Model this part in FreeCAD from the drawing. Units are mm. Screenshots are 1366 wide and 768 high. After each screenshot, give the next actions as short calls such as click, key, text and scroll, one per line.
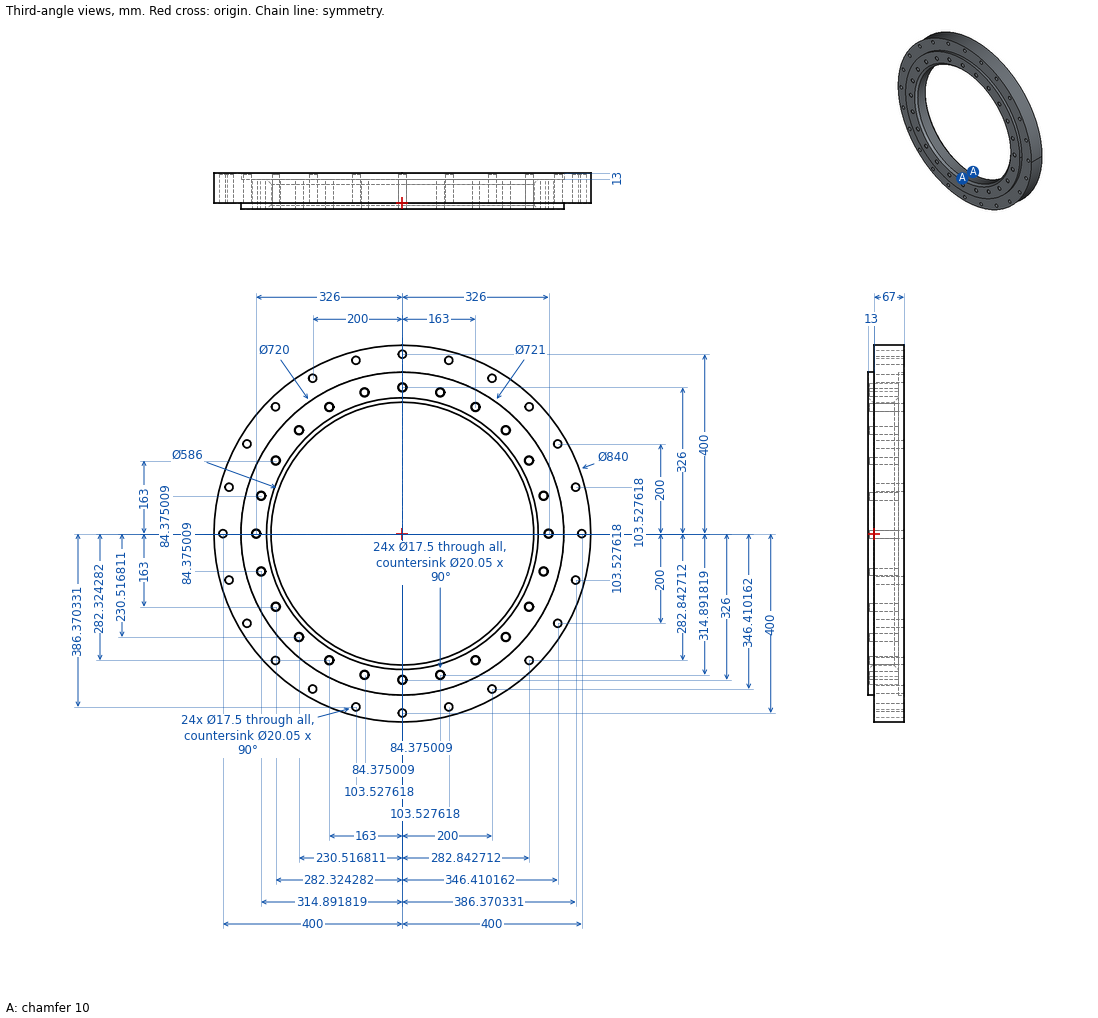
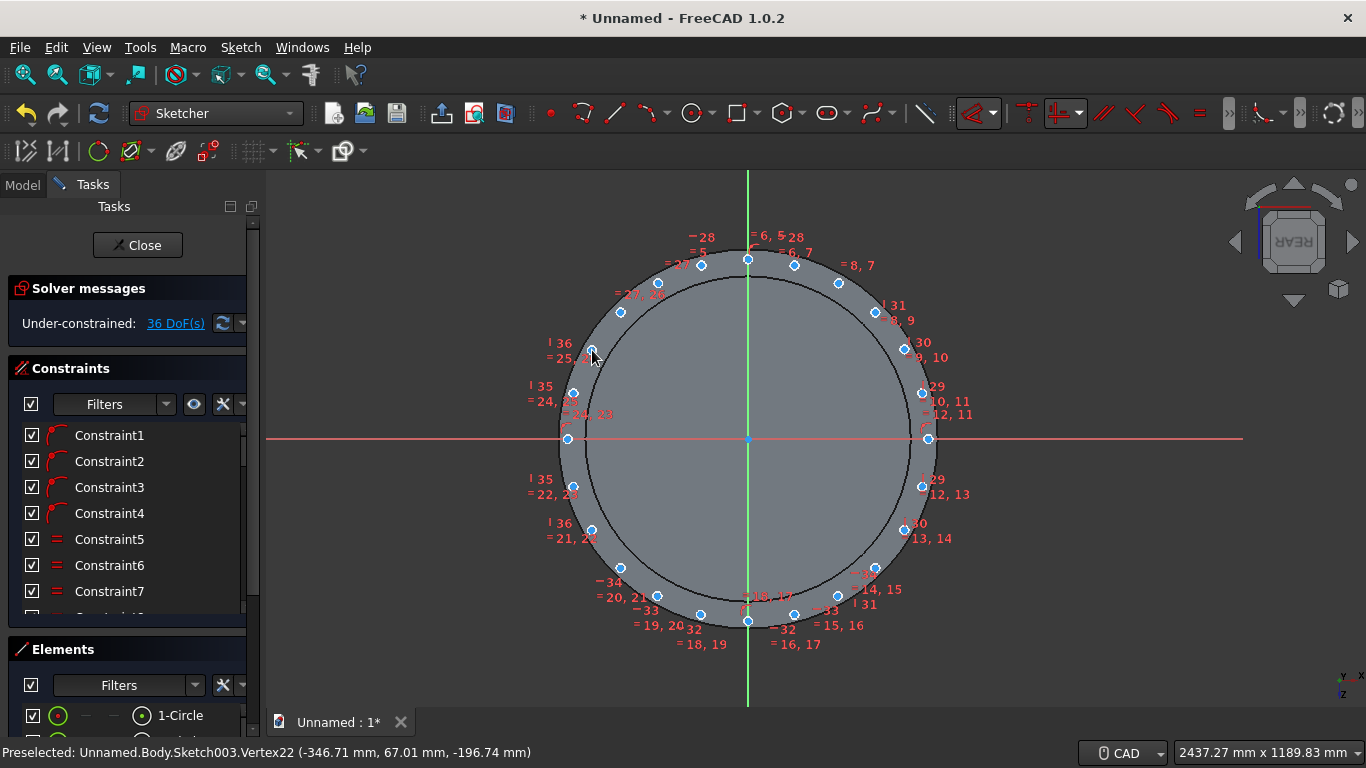
click(839, 283)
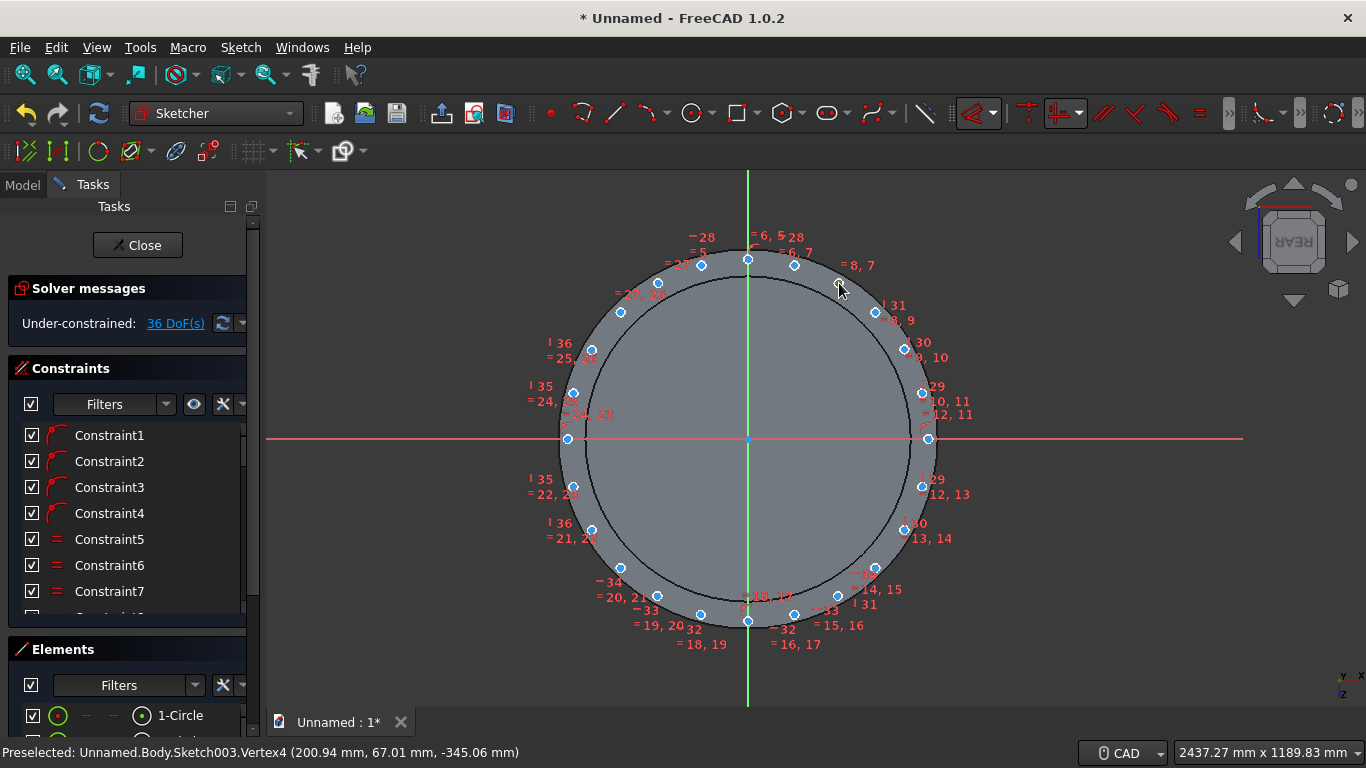
click(838, 596)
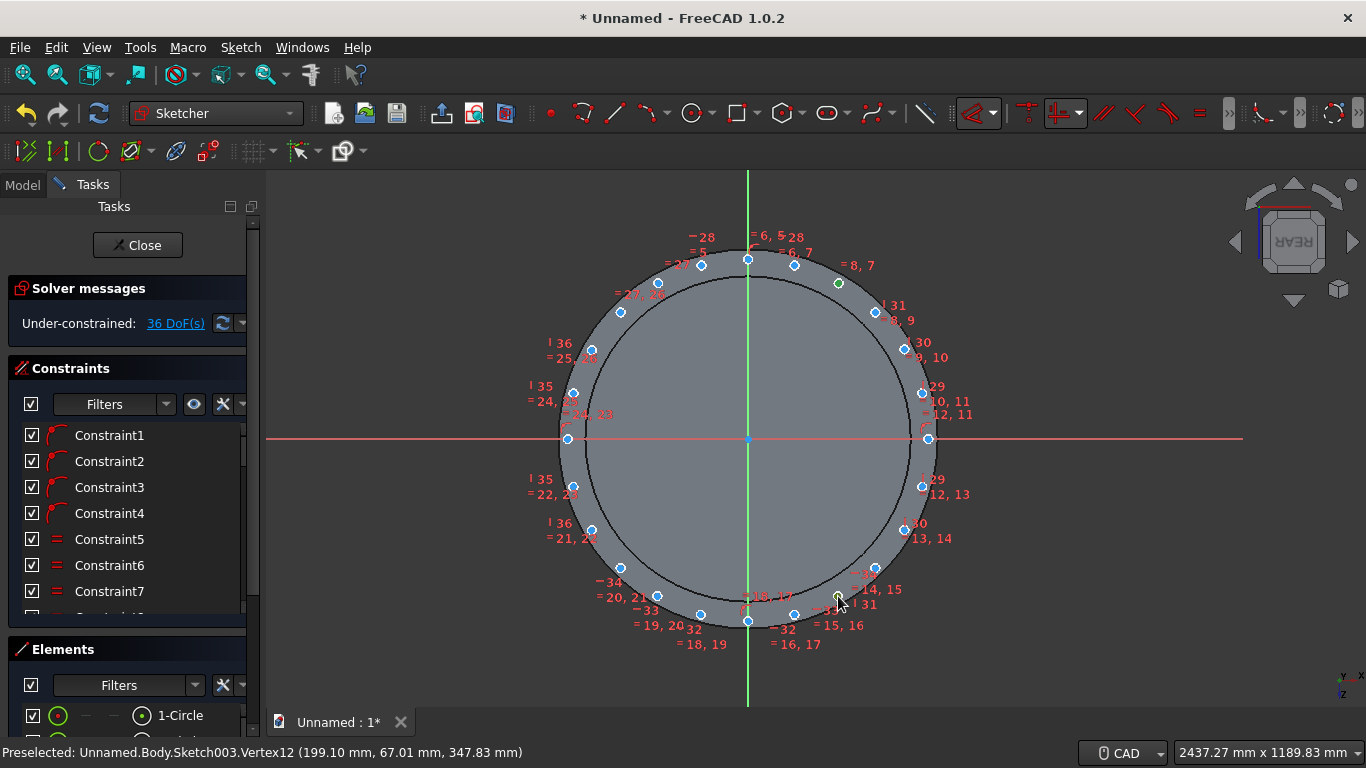
click(359, 439)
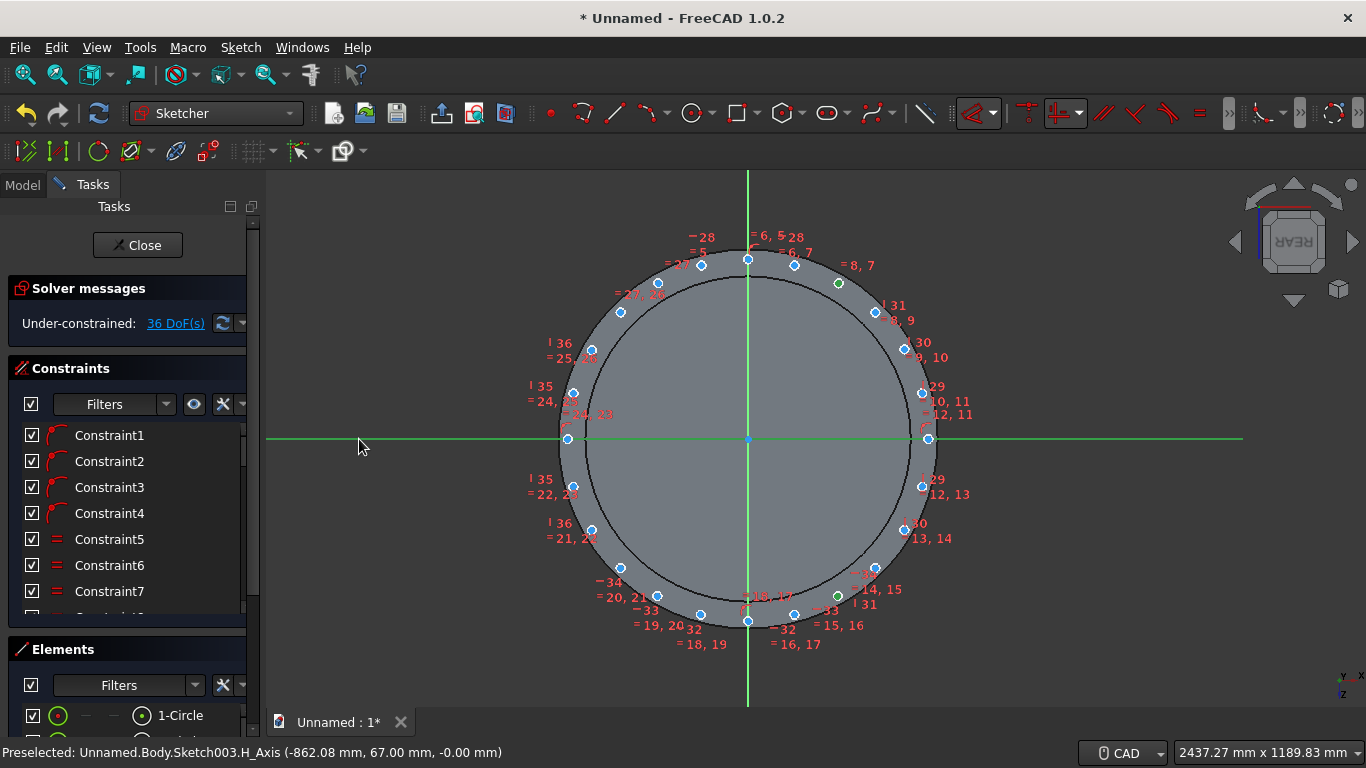
key(s)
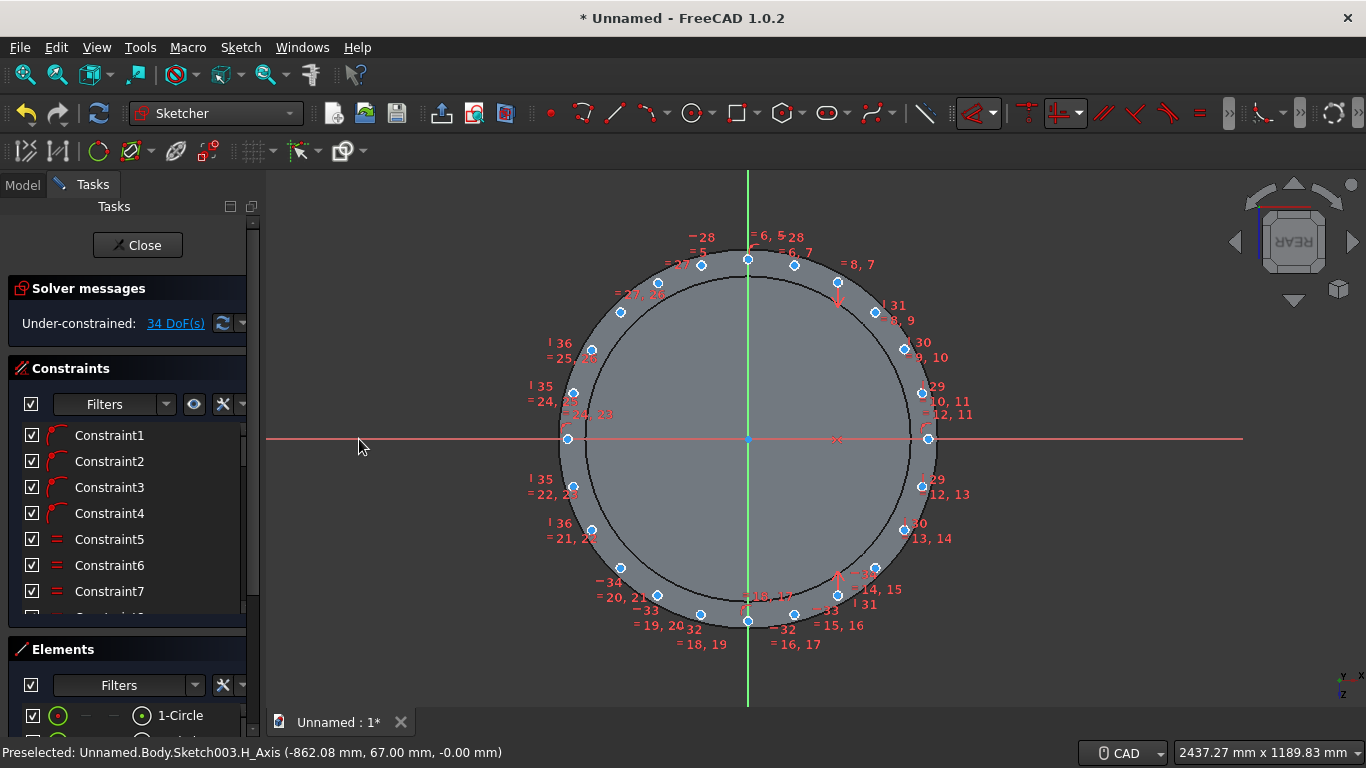
click(795, 266)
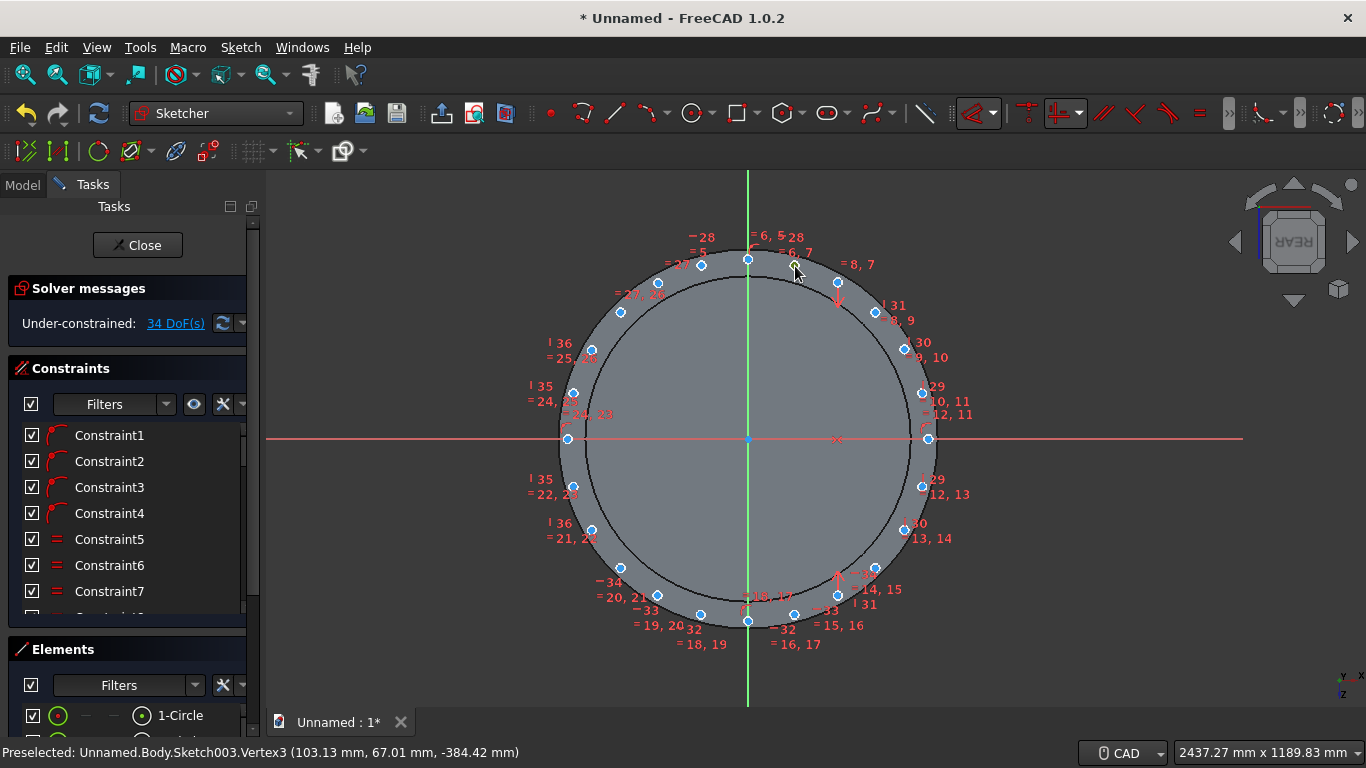
click(794, 615)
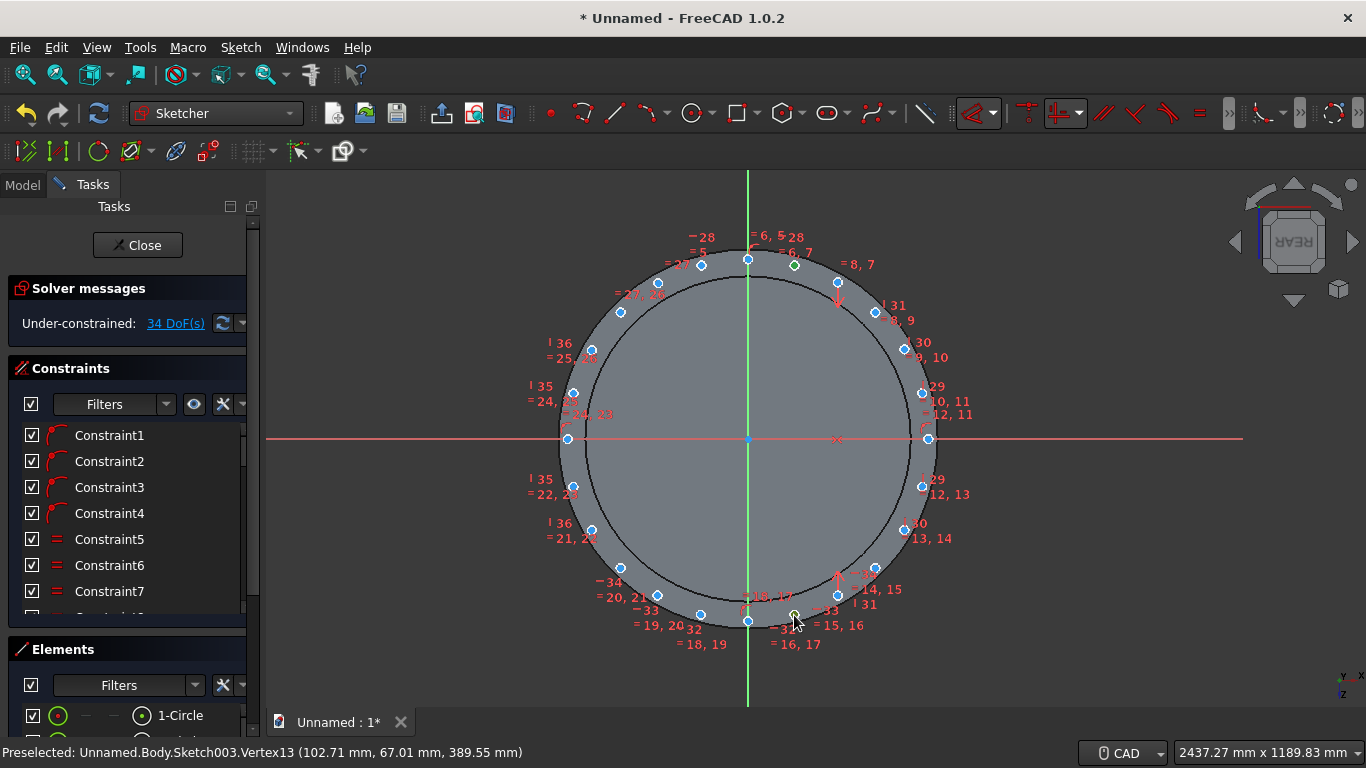
click(359, 439)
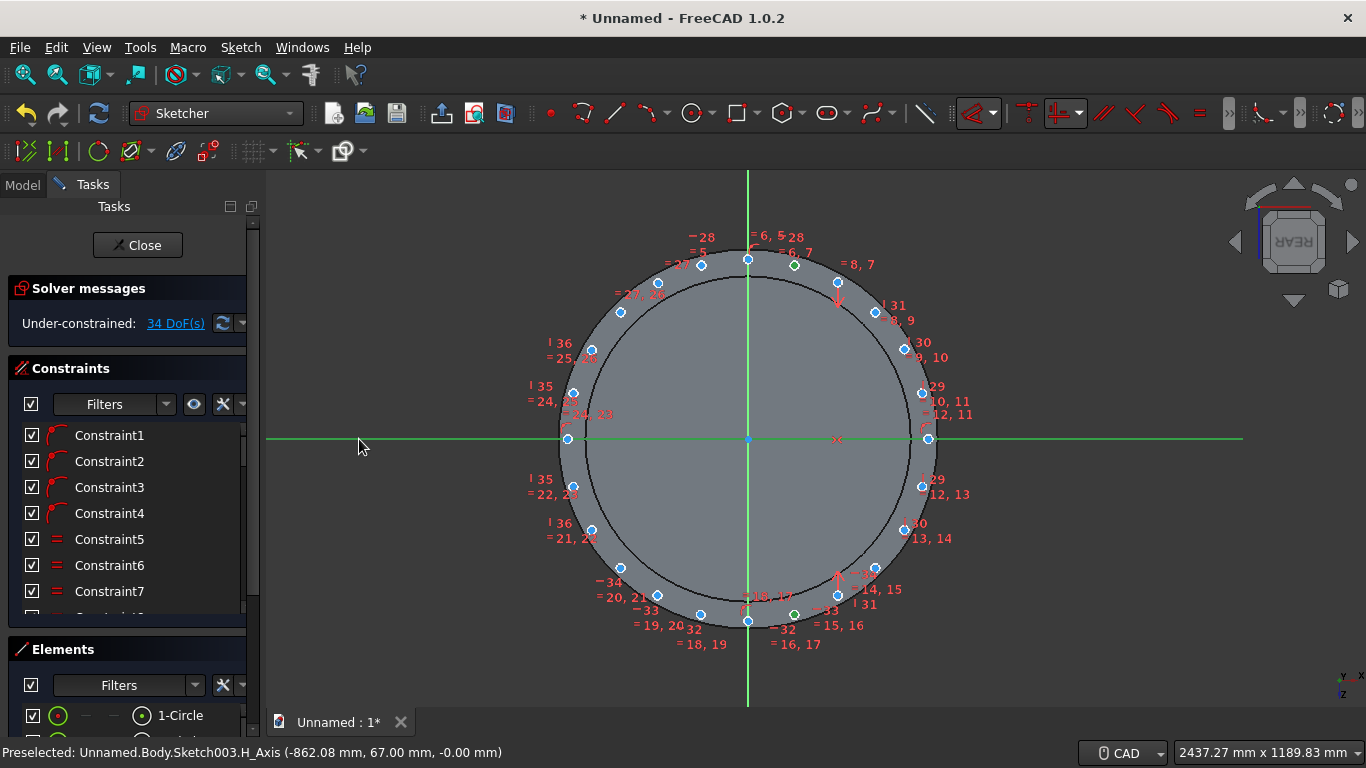
key(s)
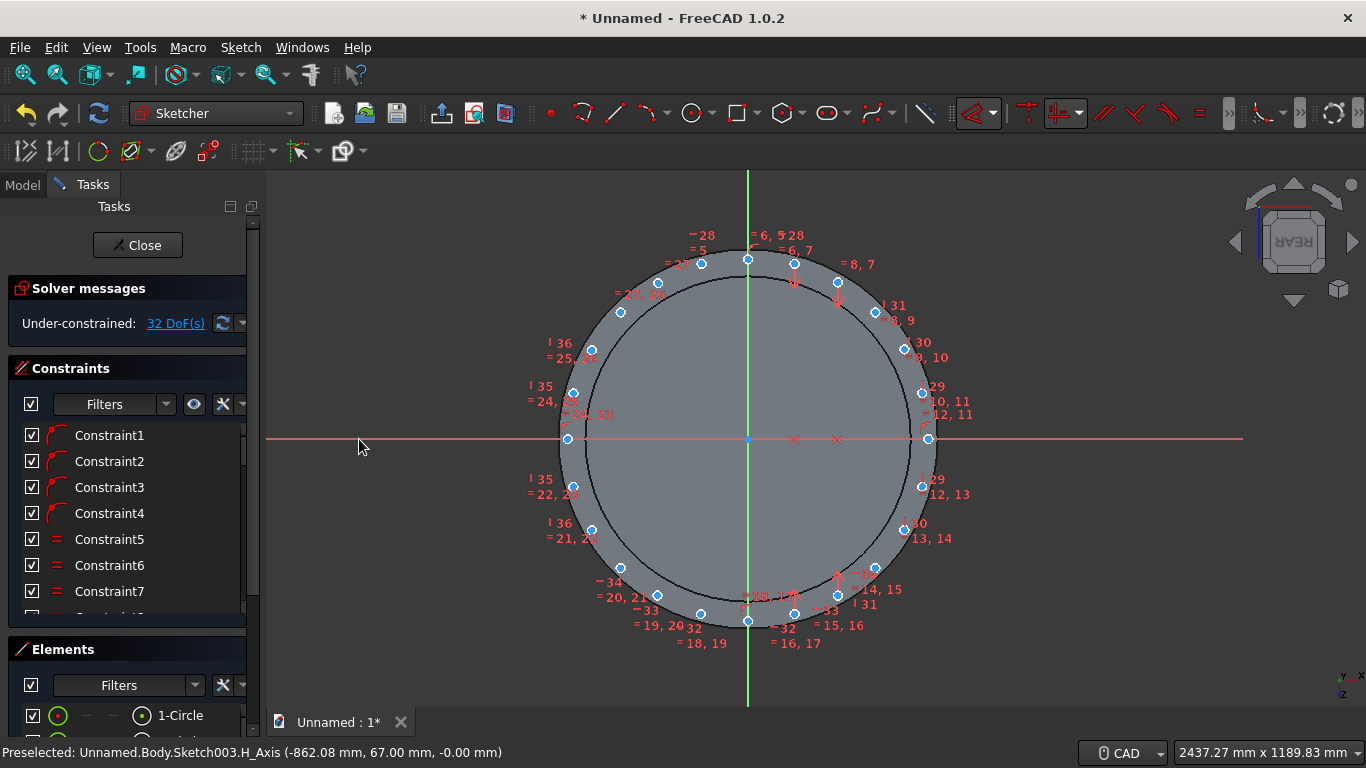
scroll(904, 530, up, 4)